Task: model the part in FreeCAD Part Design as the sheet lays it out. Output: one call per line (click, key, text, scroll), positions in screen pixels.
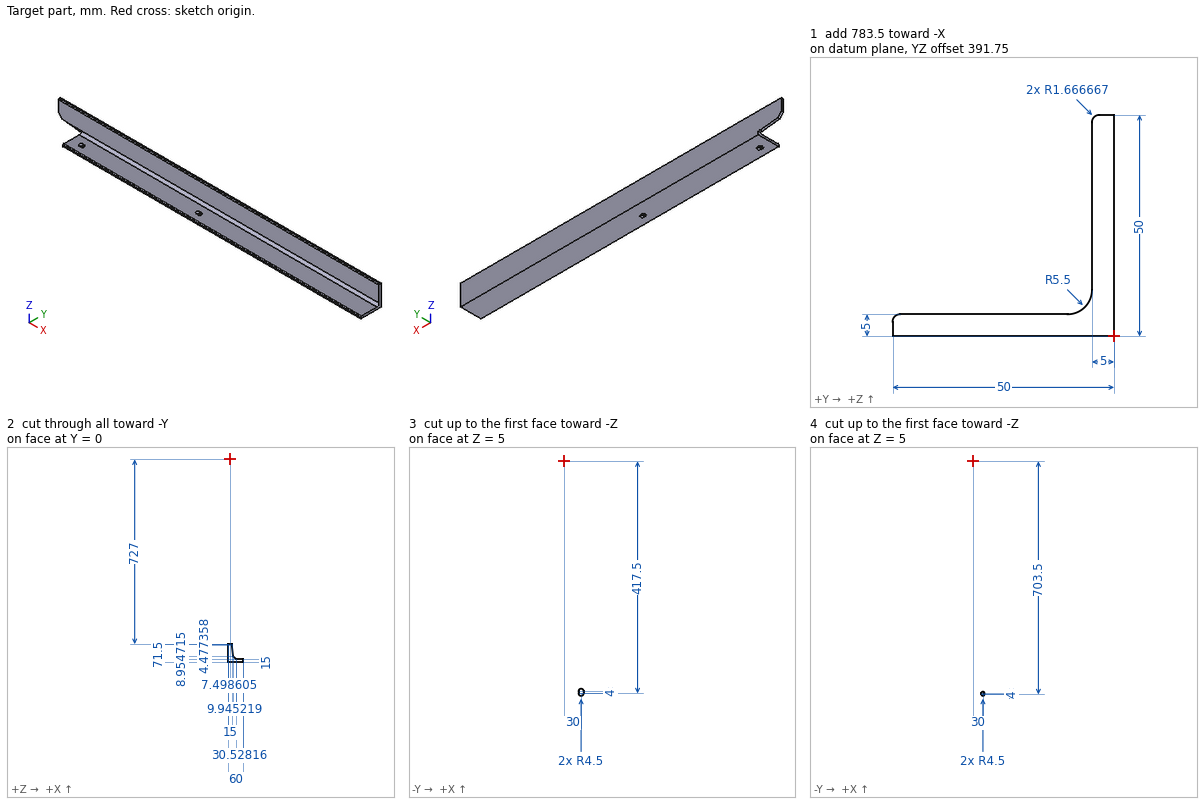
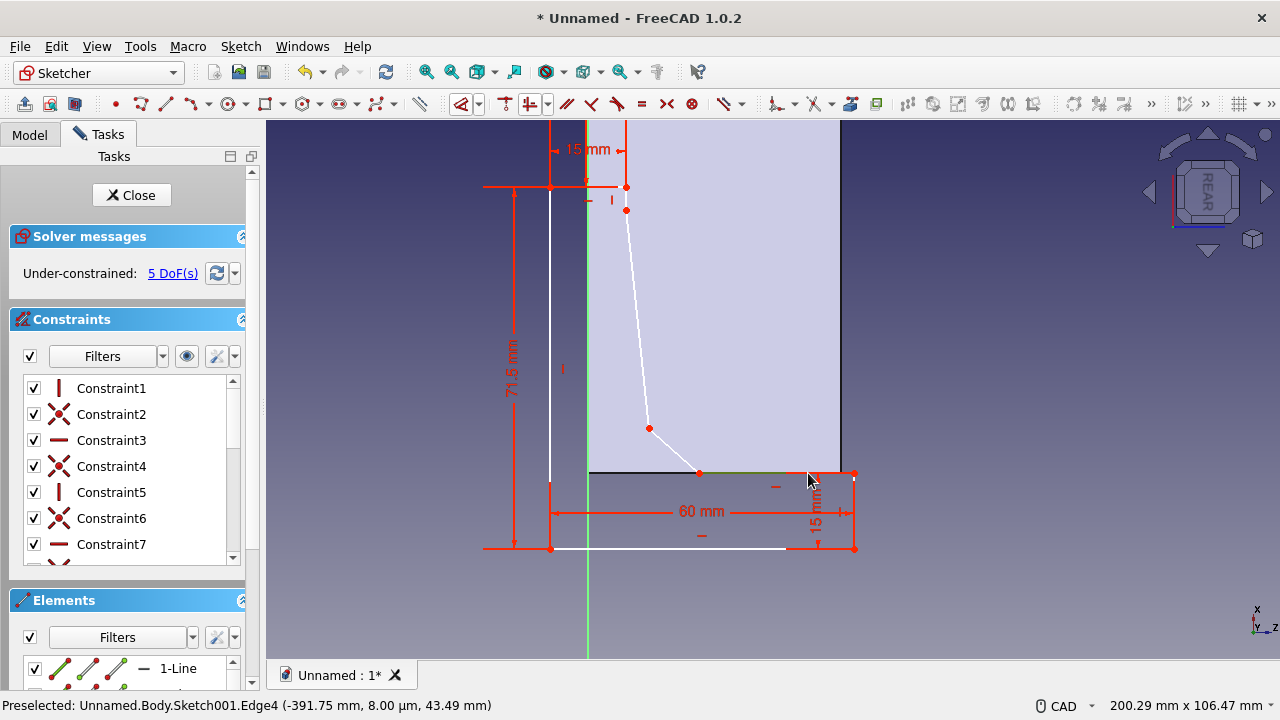
key(l)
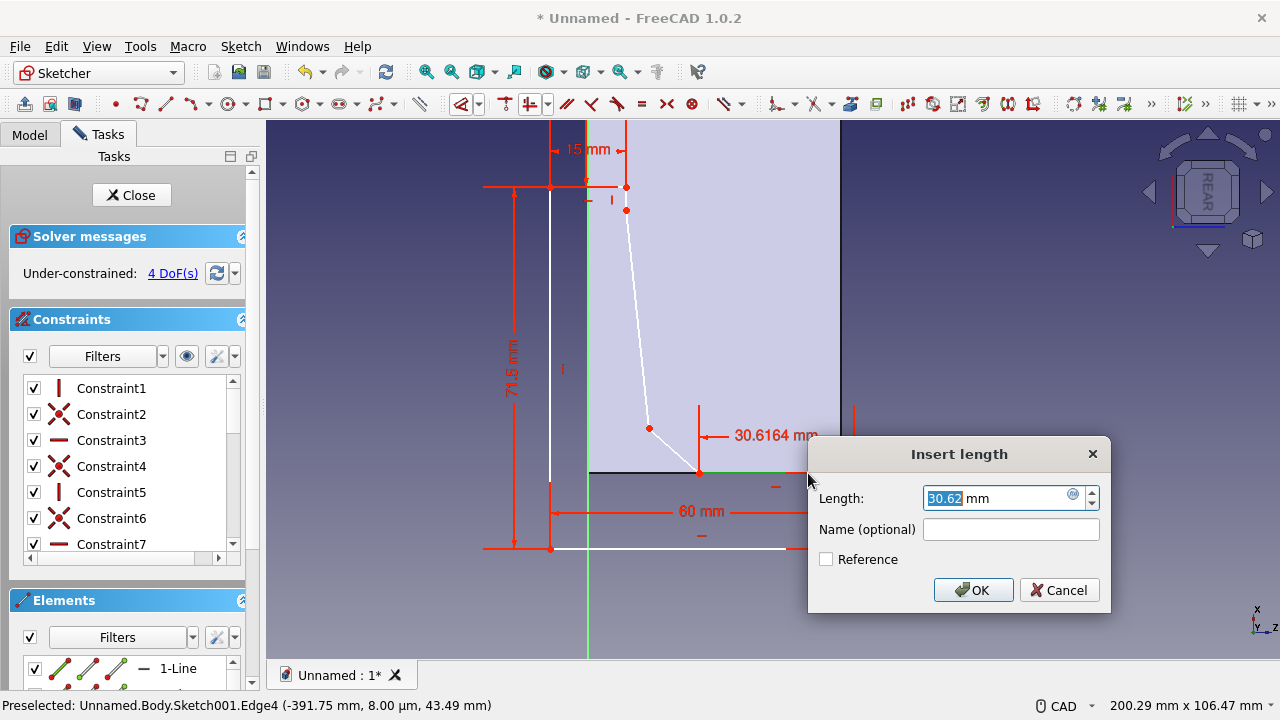
text(30.52816)
key(Return)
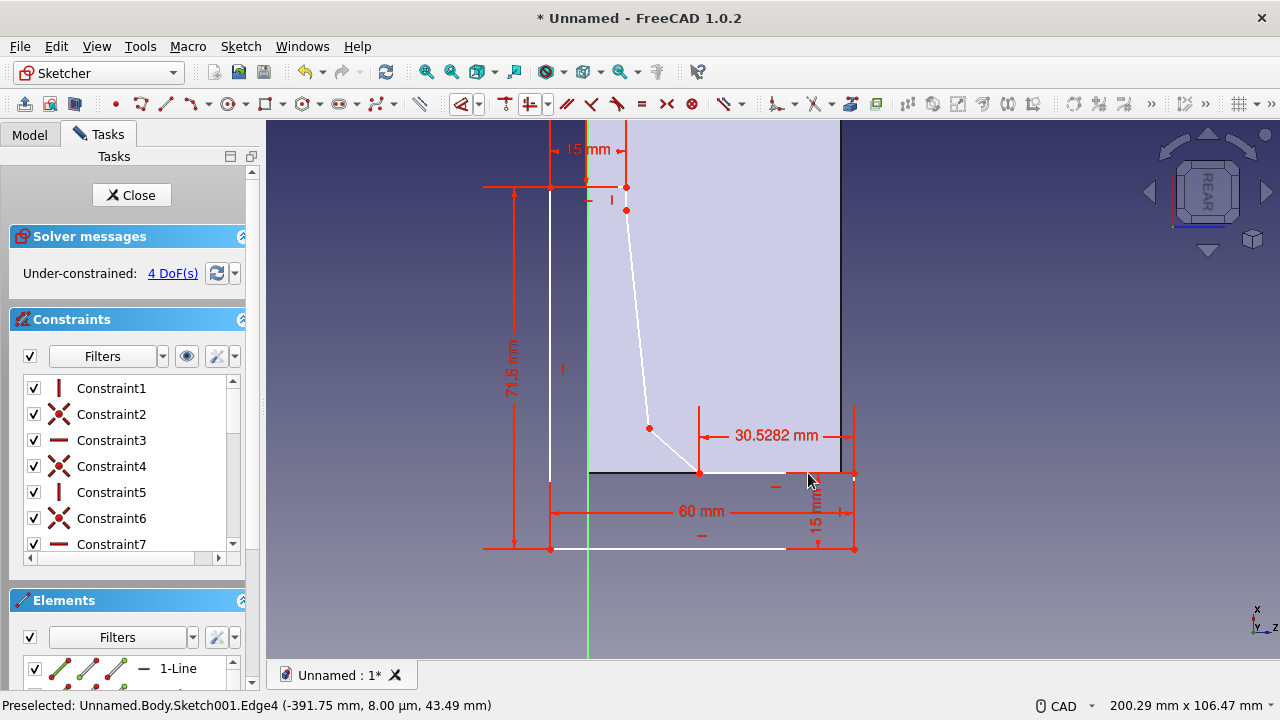
scroll(626, 202, up, 3)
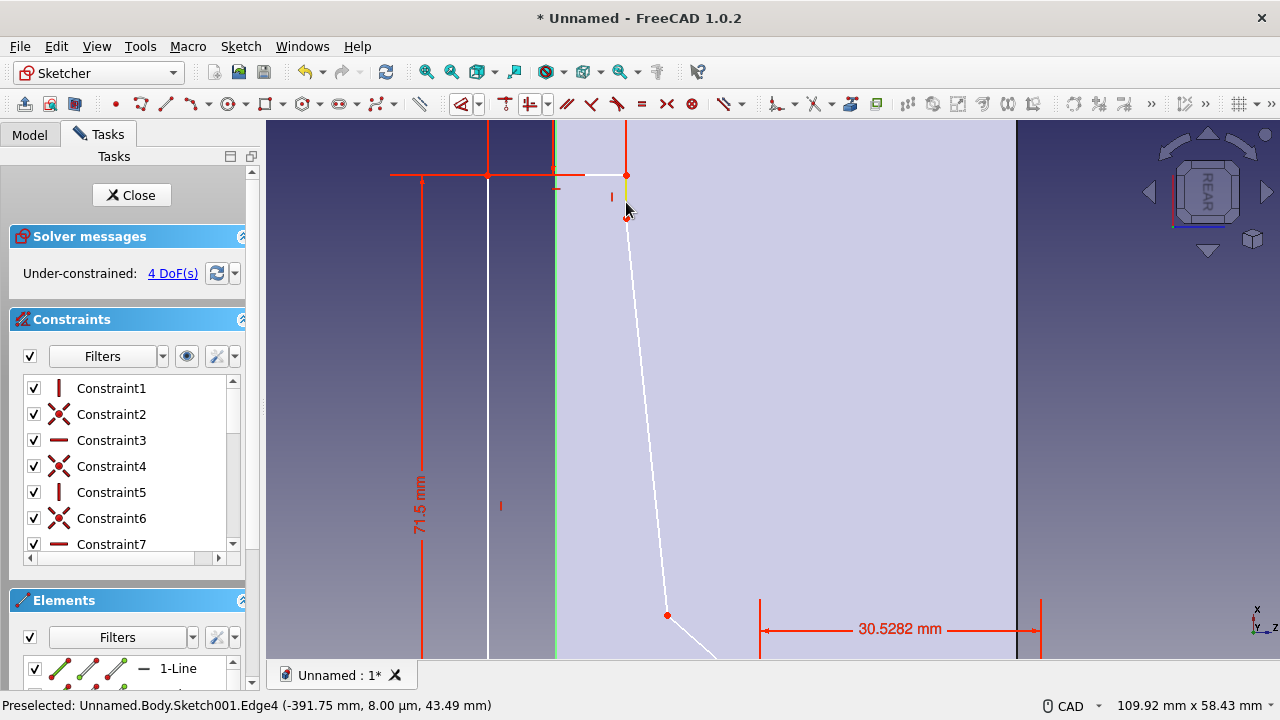
click(626, 201)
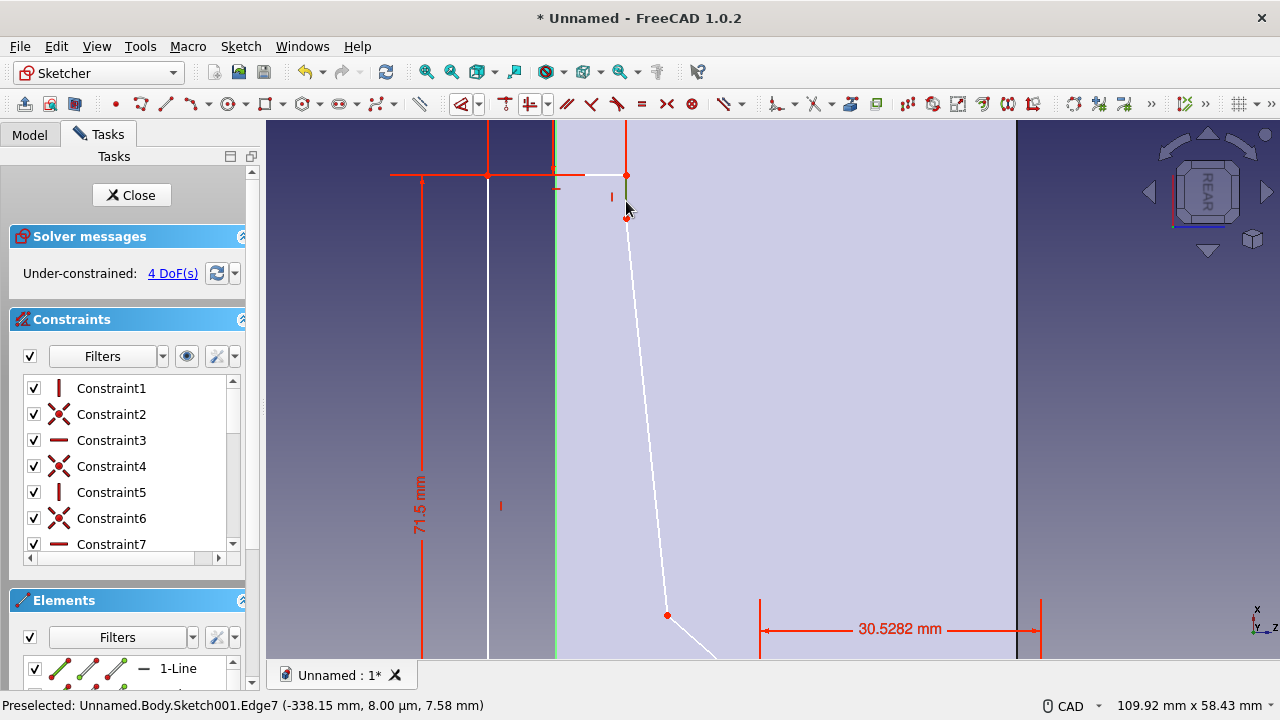
key(i)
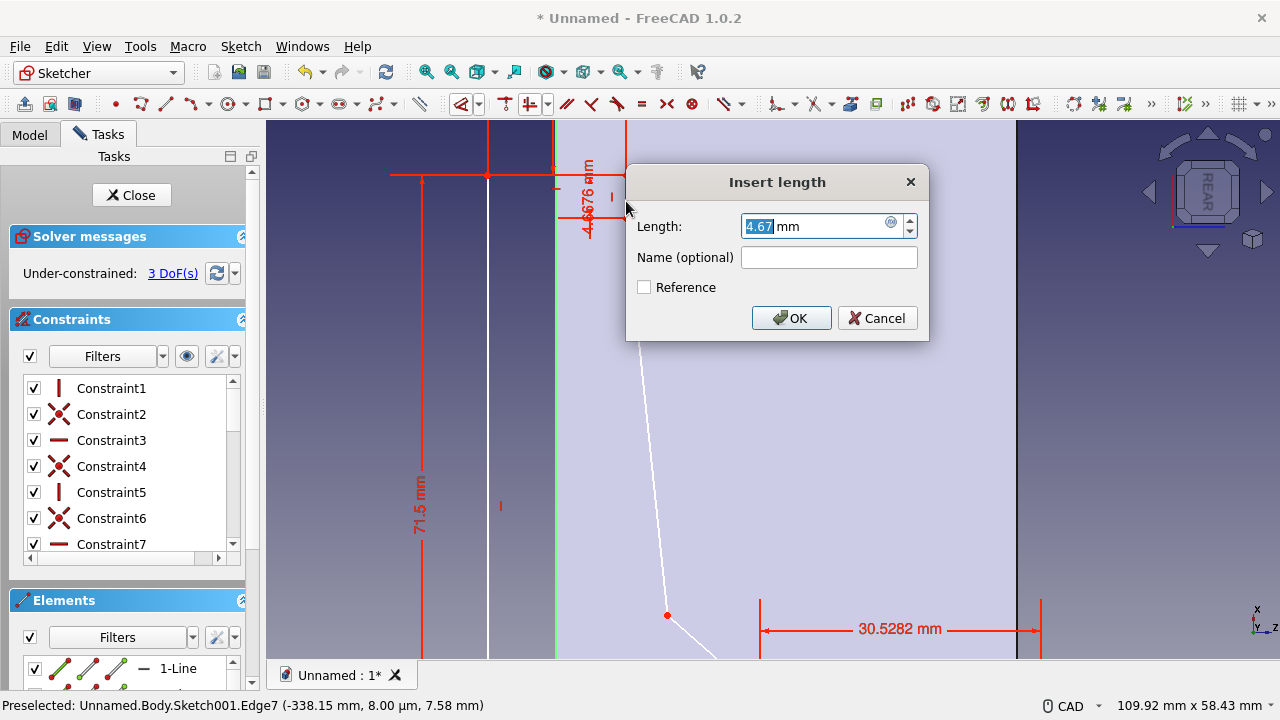
text(4.477358)
key(Return)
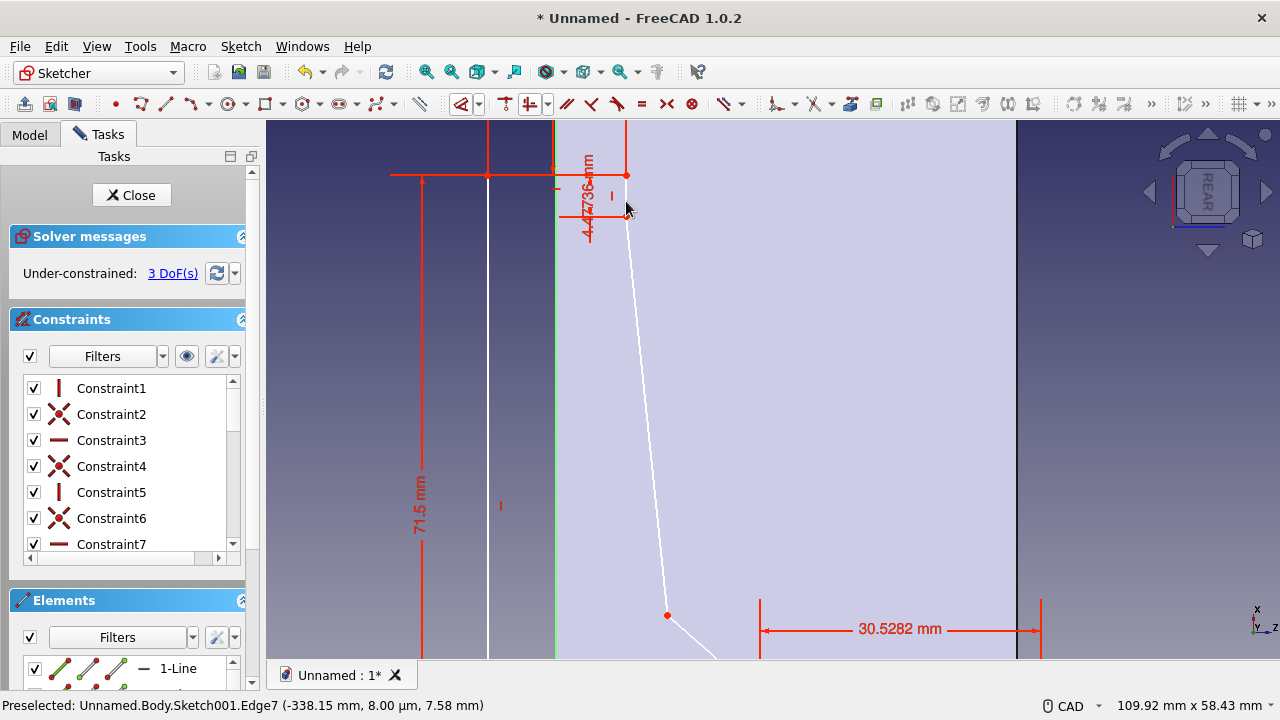
click(488, 175)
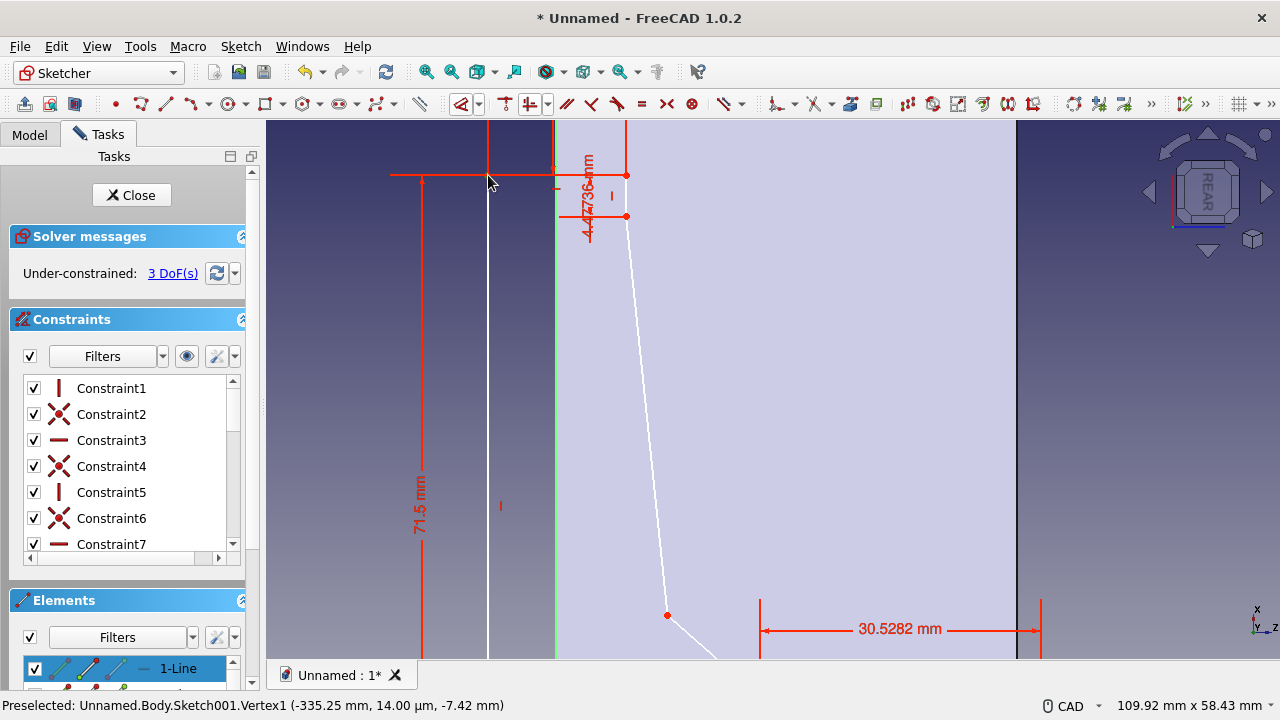
click(478, 104)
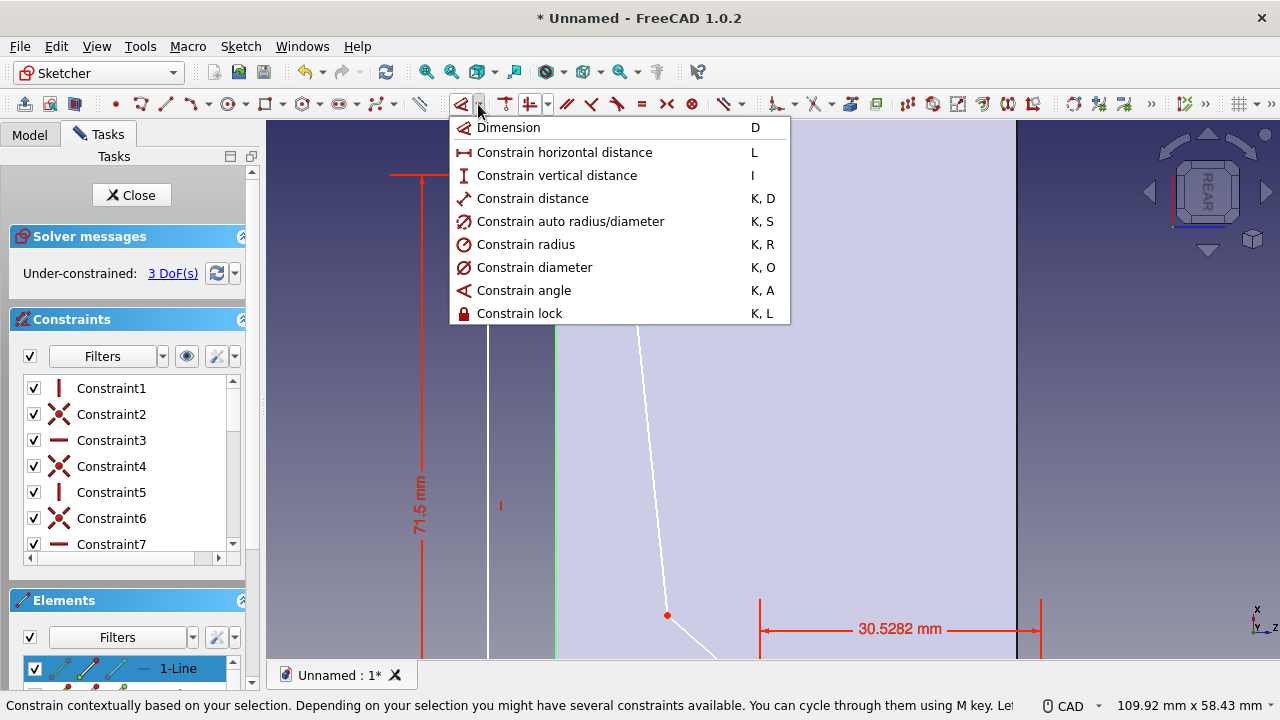
click(620, 152)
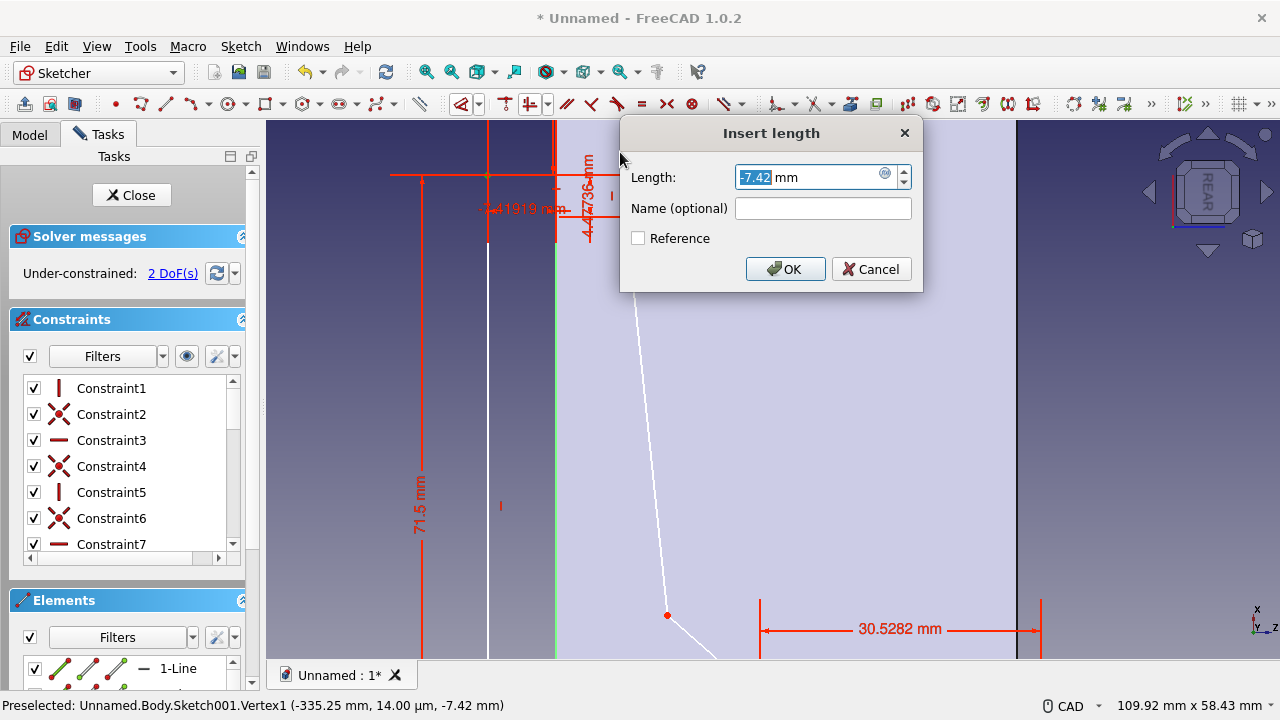
text(-7.498605)
key(Return)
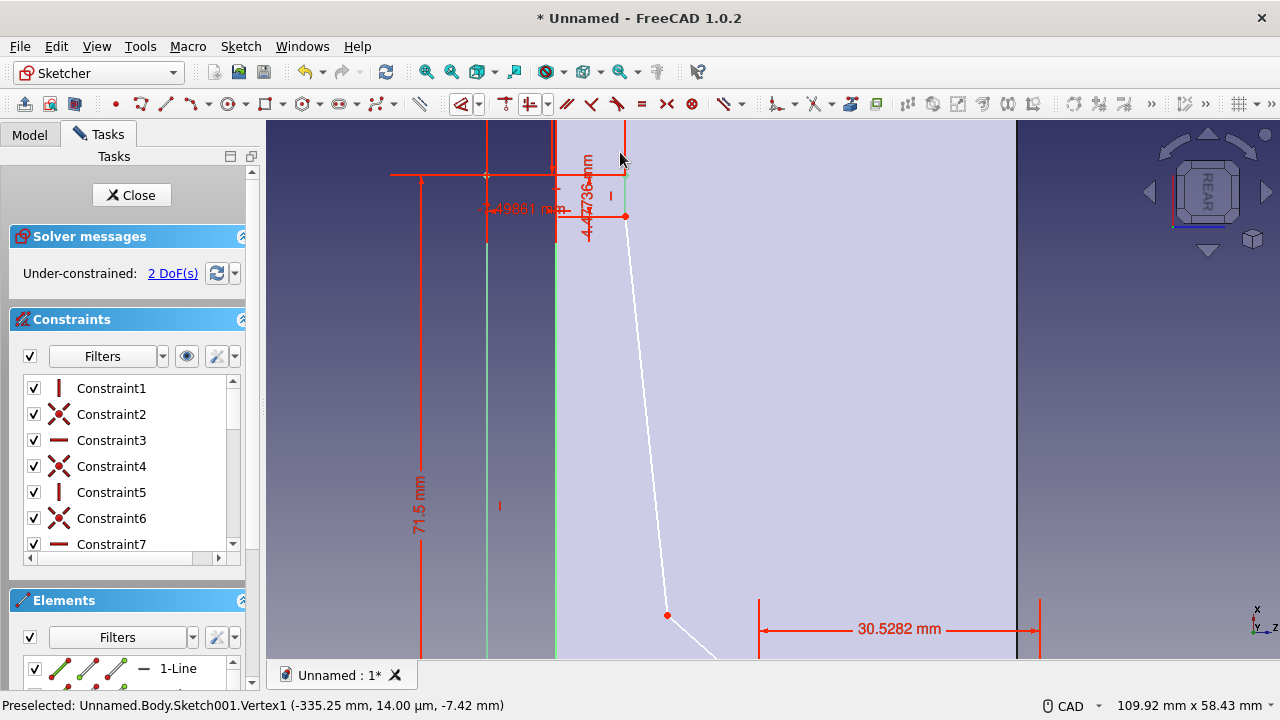
scroll(633, 249, down, 3)